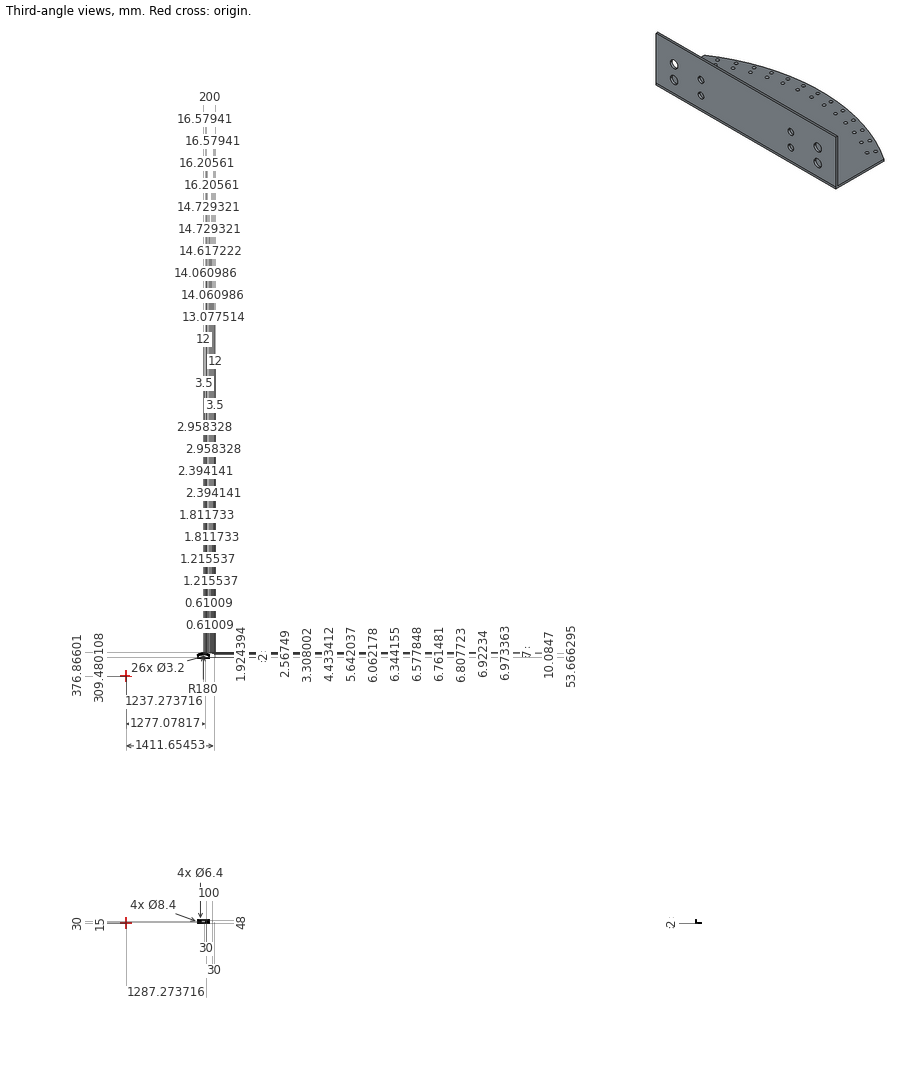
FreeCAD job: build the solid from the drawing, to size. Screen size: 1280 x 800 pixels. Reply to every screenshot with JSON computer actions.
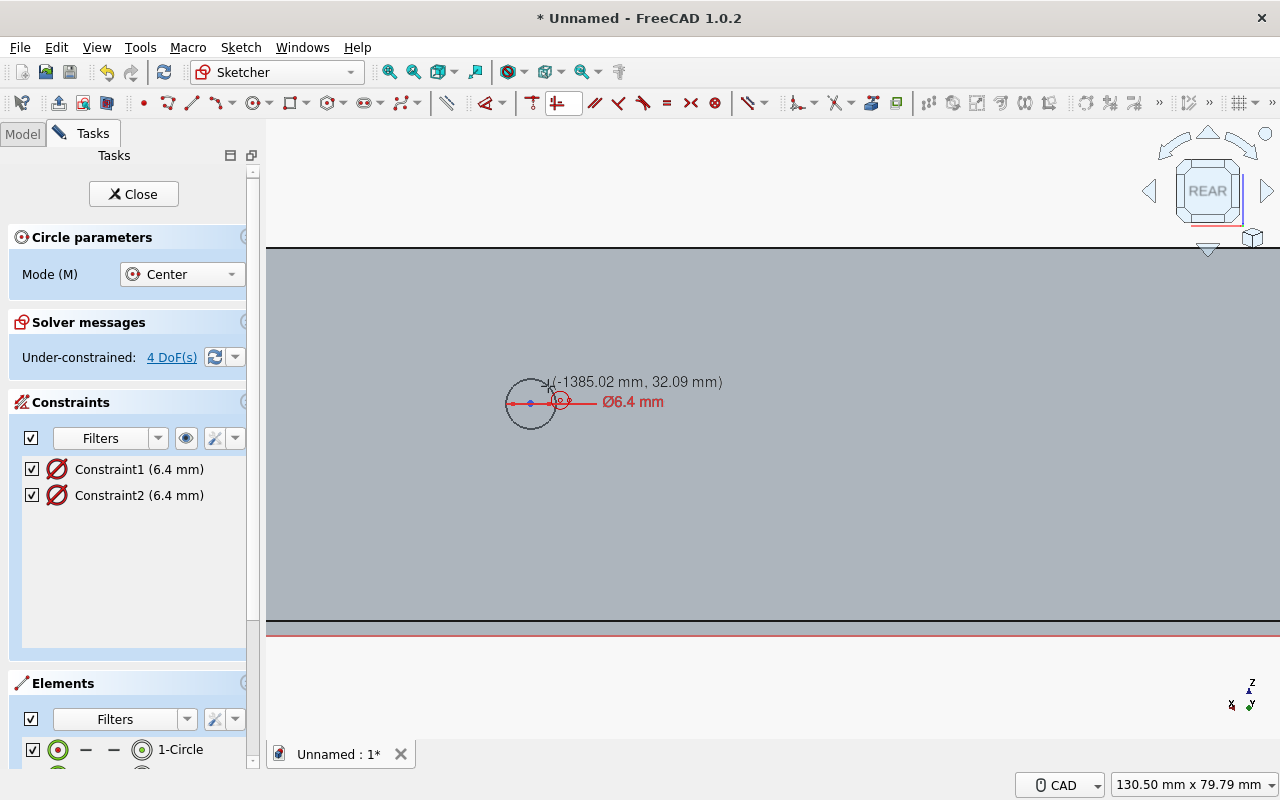
{"action": "scroll", "coordinate": [529, 402], "scroll_direction": "down", "scroll_amount": 4}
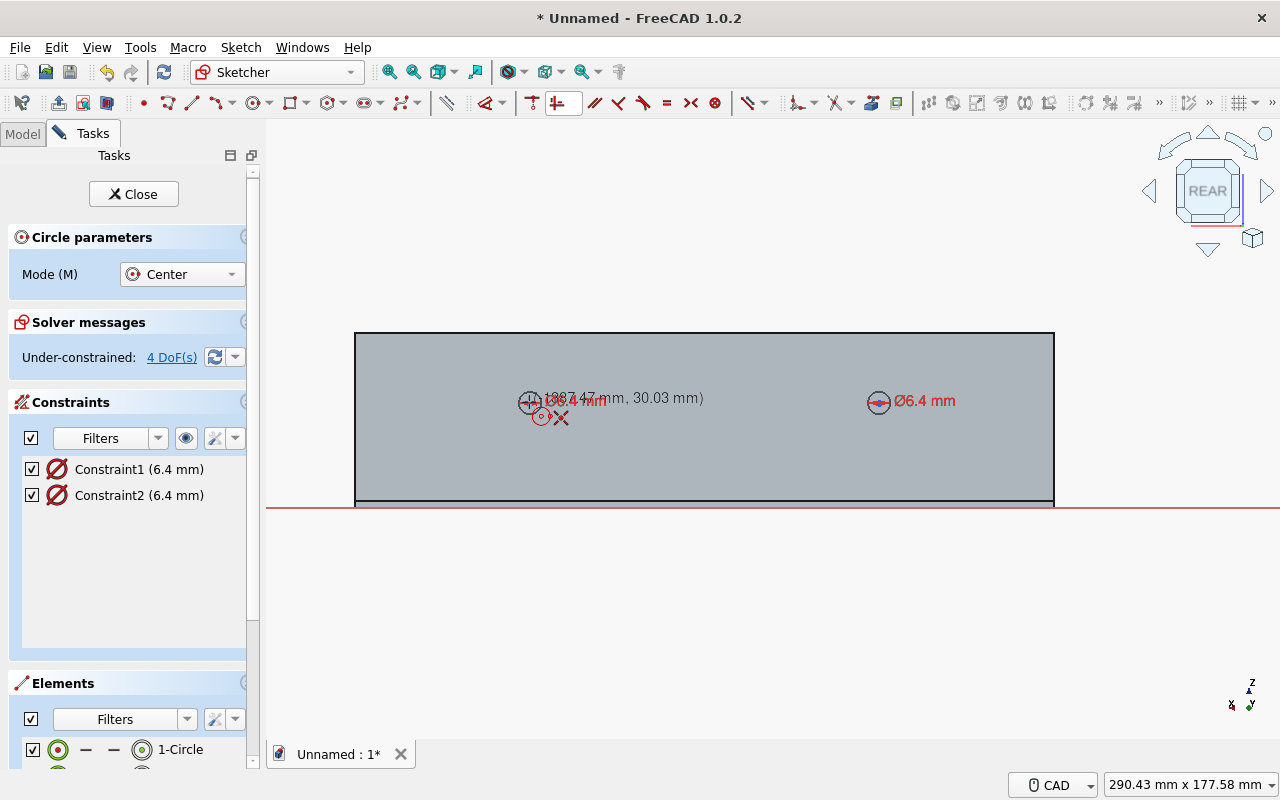
{"action": "scroll", "coordinate": [984, 455], "scroll_direction": "up", "scroll_amount": 3}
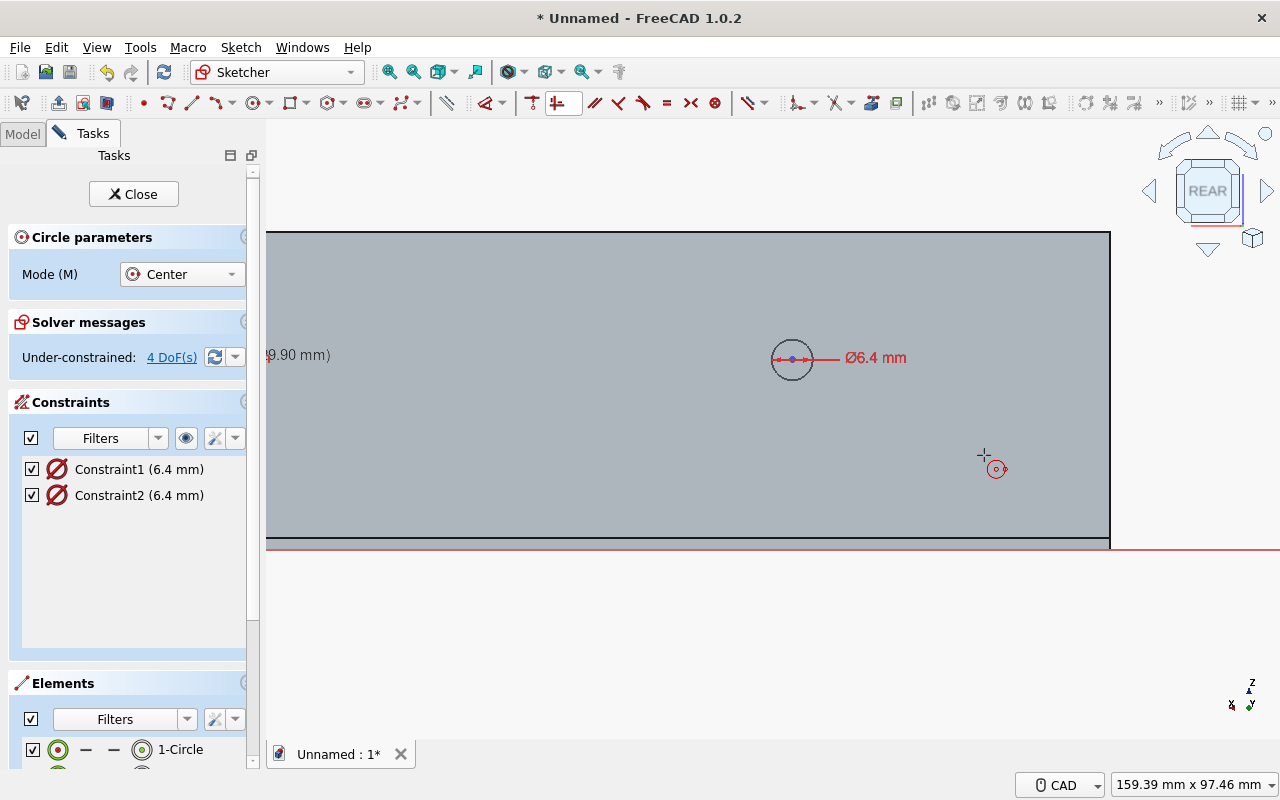
{"action": "left_click", "coordinate": [983, 455]}
{"action": "mouse_move", "coordinate": [1002, 436]}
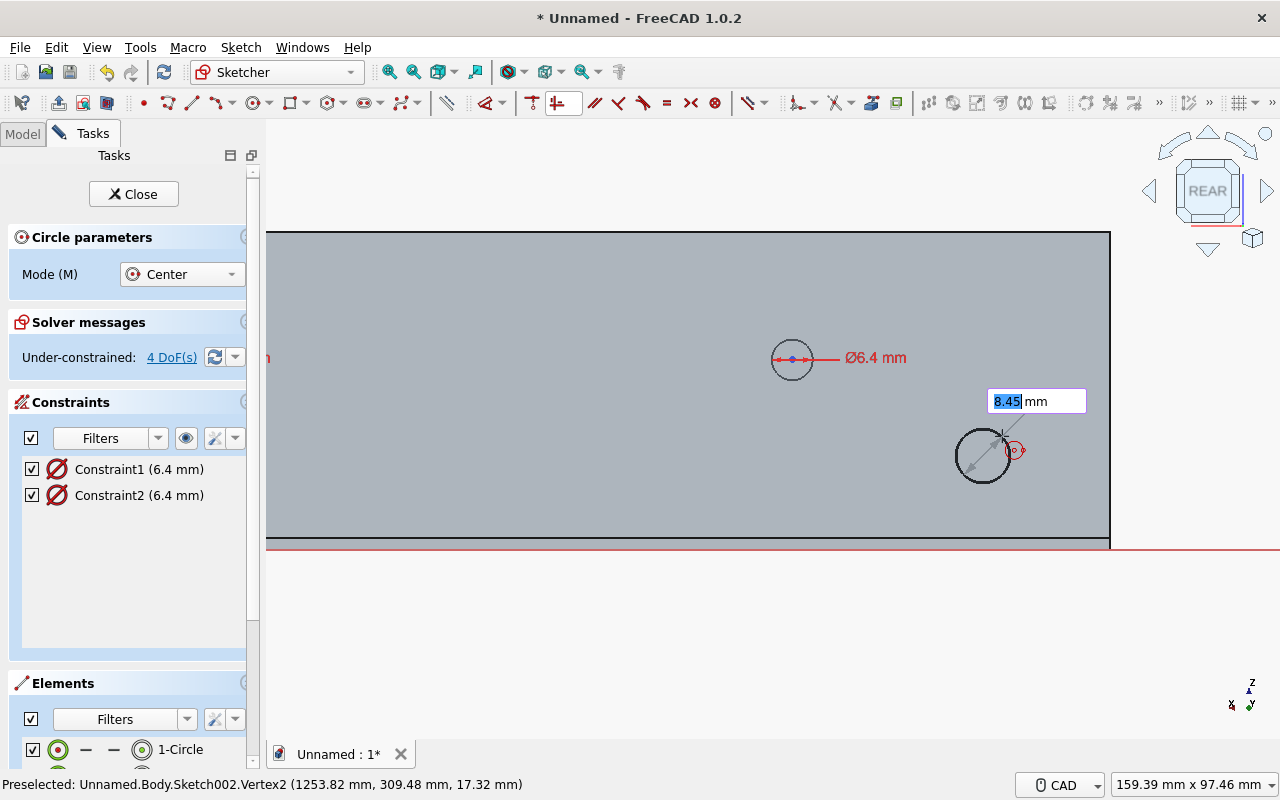
{"action": "type", "text": "8.4"}
{"action": "key", "text": "Return"}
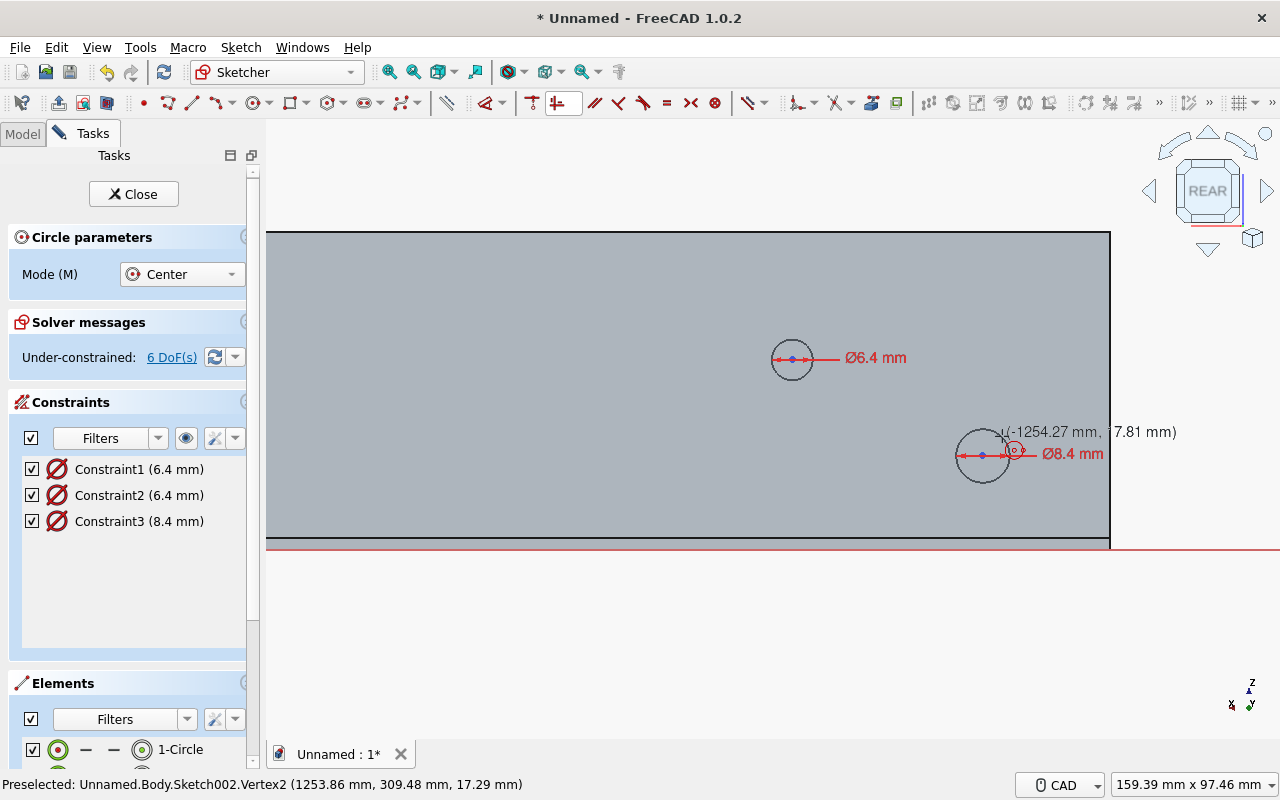
{"action": "scroll", "coordinate": [985, 456], "scroll_direction": "down", "scroll_amount": 3}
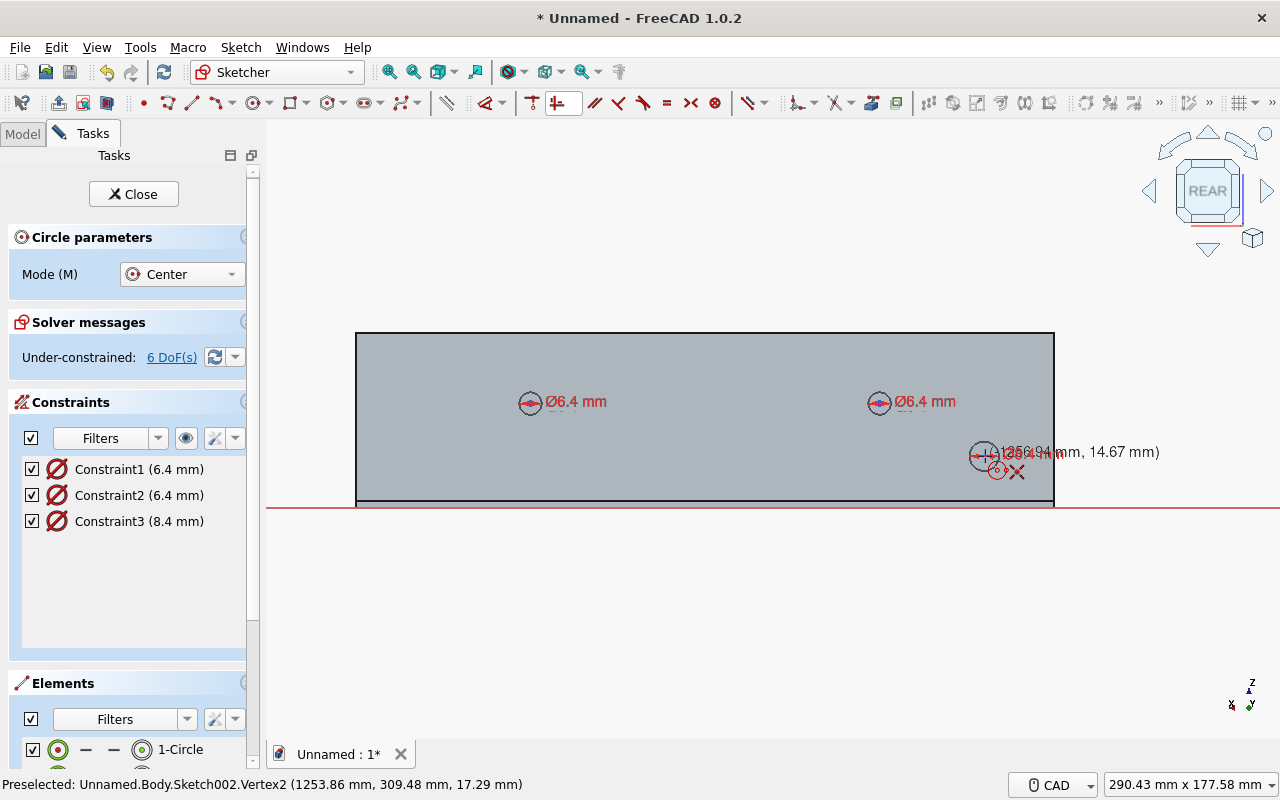
{"action": "scroll", "coordinate": [426, 456], "scroll_direction": "up", "scroll_amount": 3}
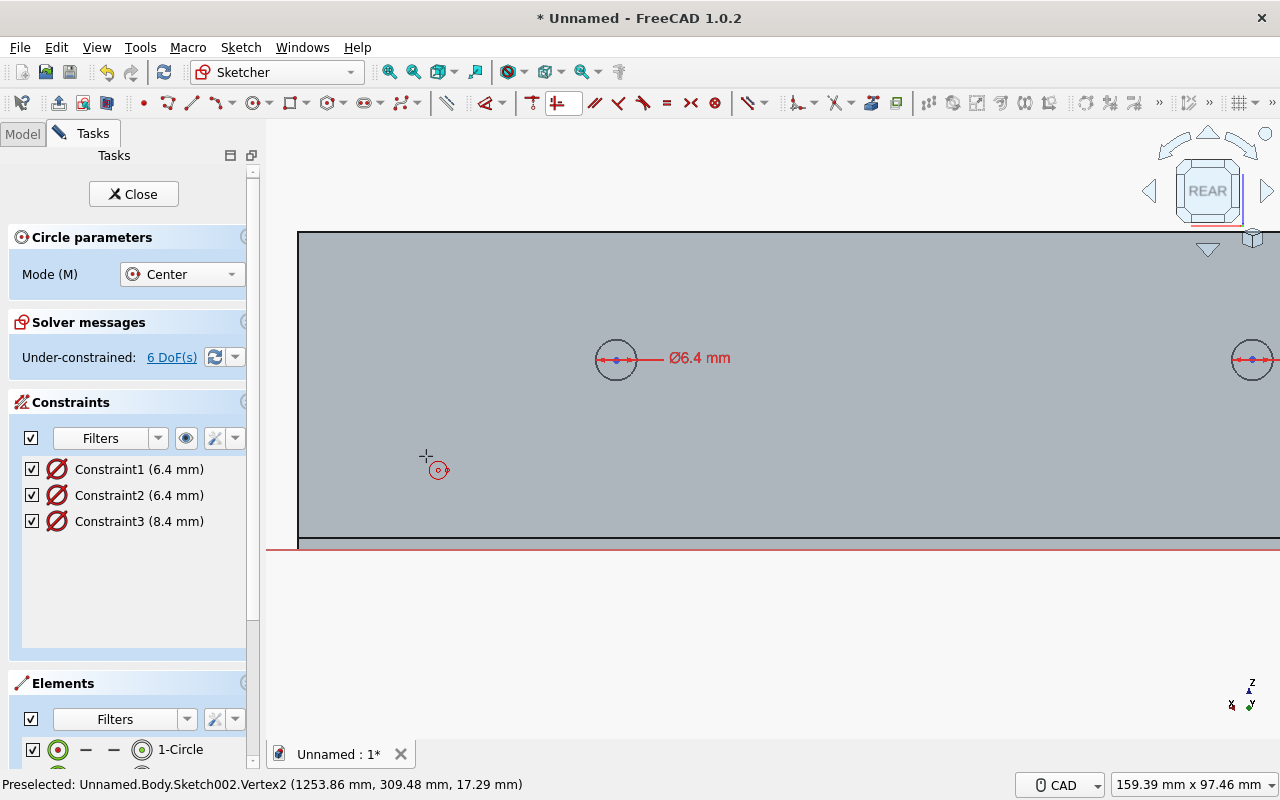
{"action": "left_click", "coordinate": [425, 455]}
{"action": "mouse_move", "coordinate": [444, 436]}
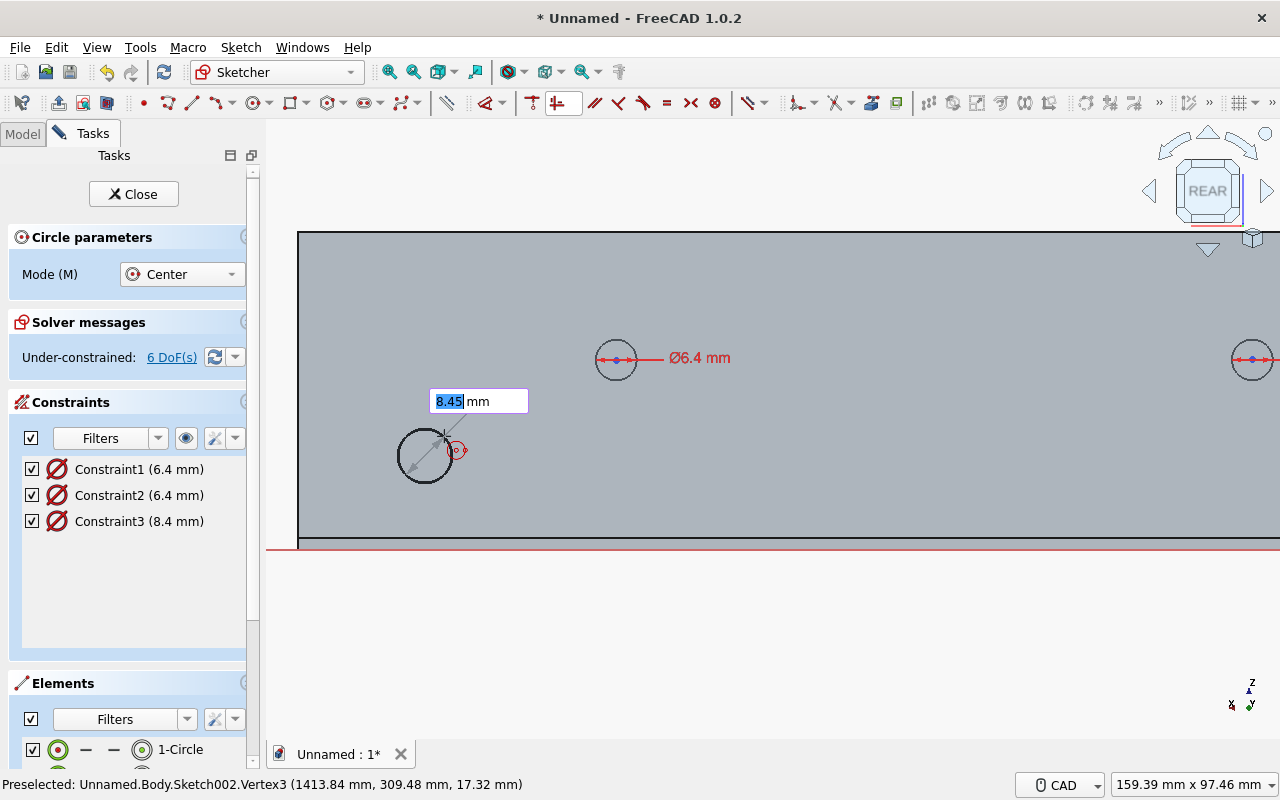
{"action": "type", "text": "8.4"}
{"action": "key", "text": "Return"}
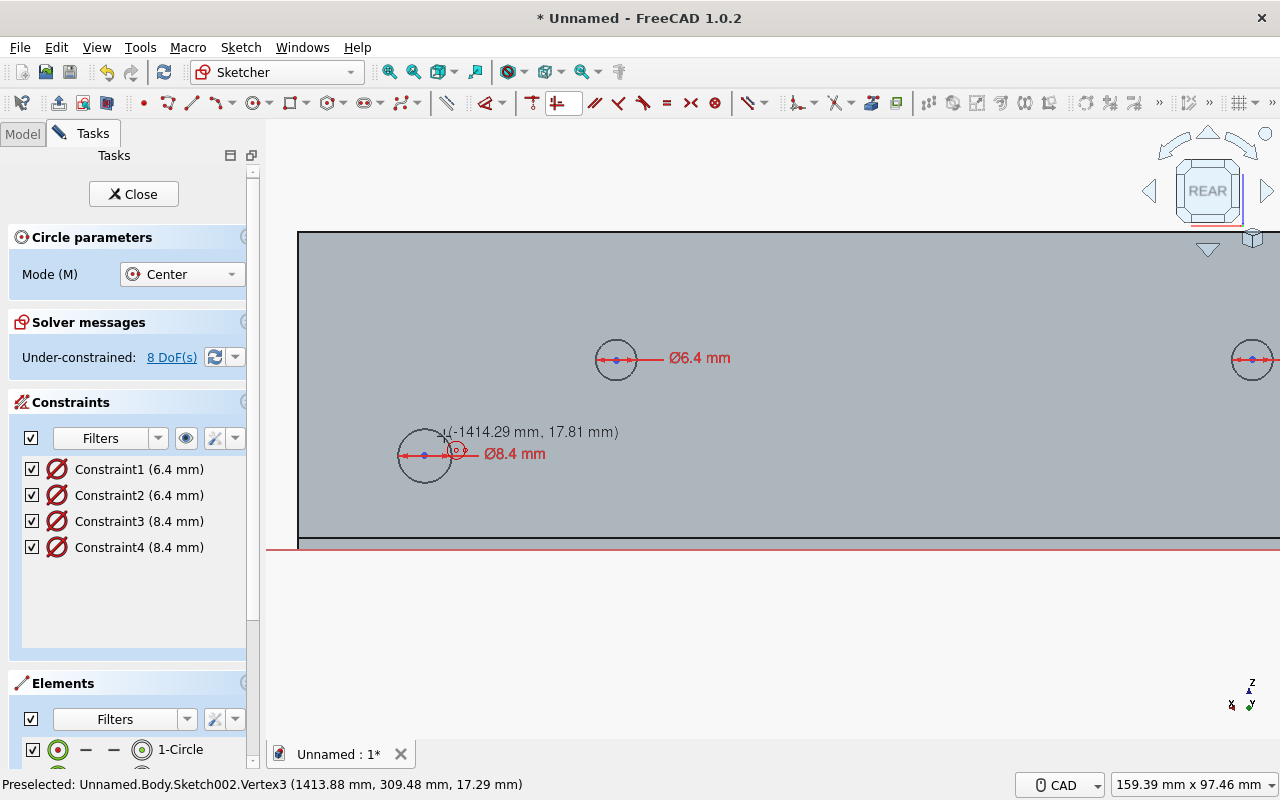
{"action": "scroll", "coordinate": [425, 456], "scroll_direction": "down", "scroll_amount": 3}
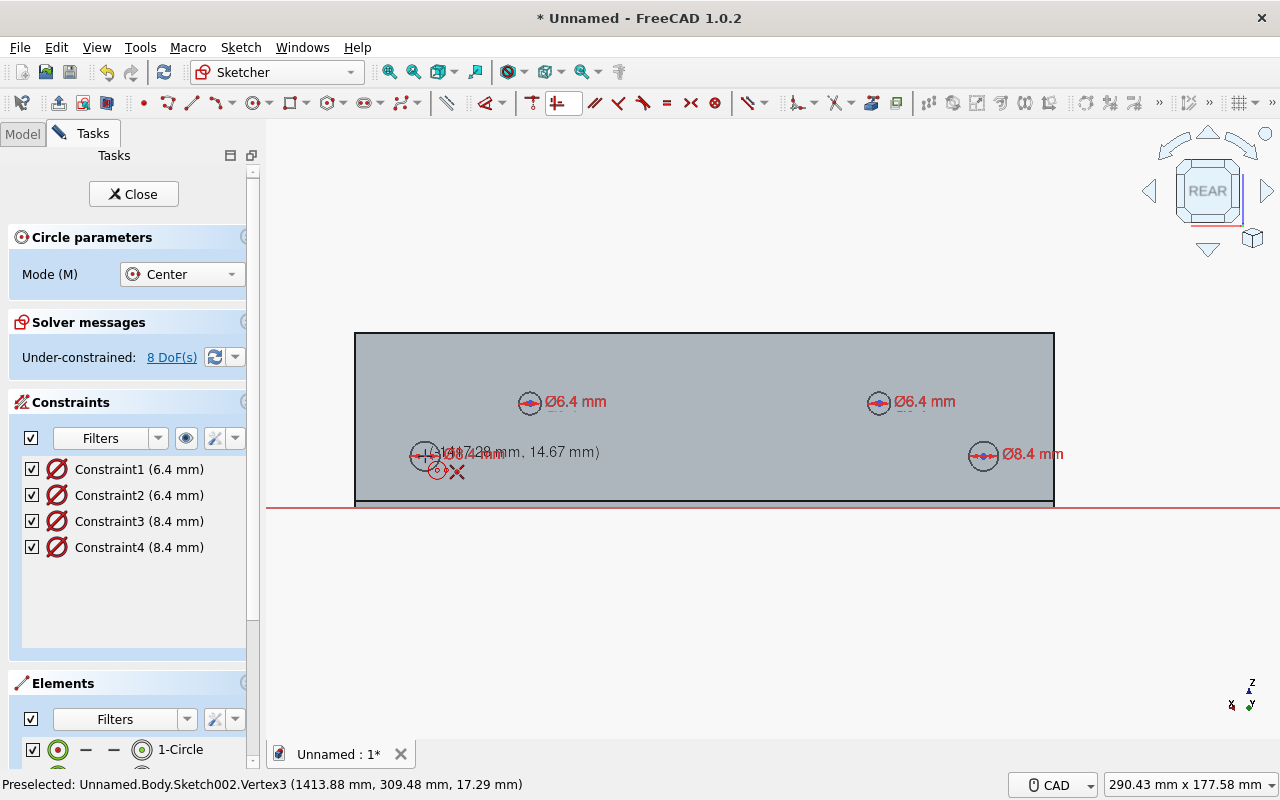
{"action": "scroll", "coordinate": [984, 403], "scroll_direction": "up", "scroll_amount": 3}